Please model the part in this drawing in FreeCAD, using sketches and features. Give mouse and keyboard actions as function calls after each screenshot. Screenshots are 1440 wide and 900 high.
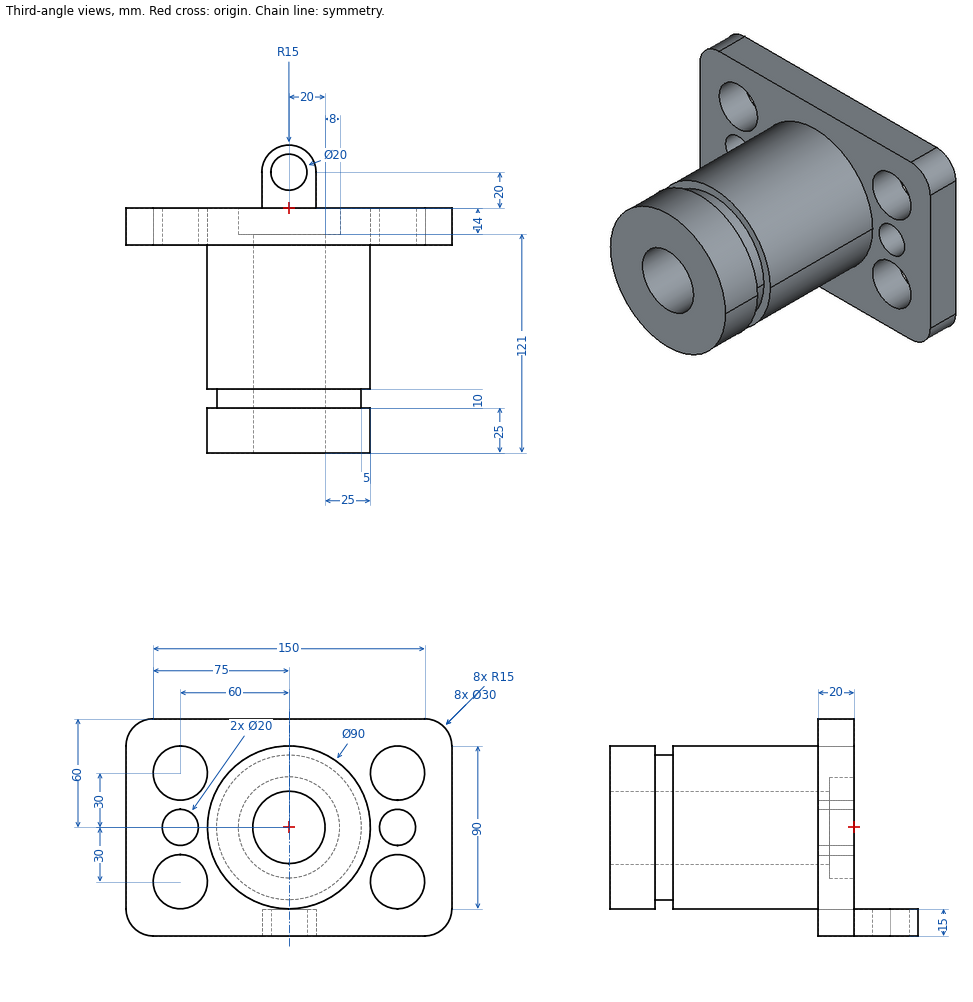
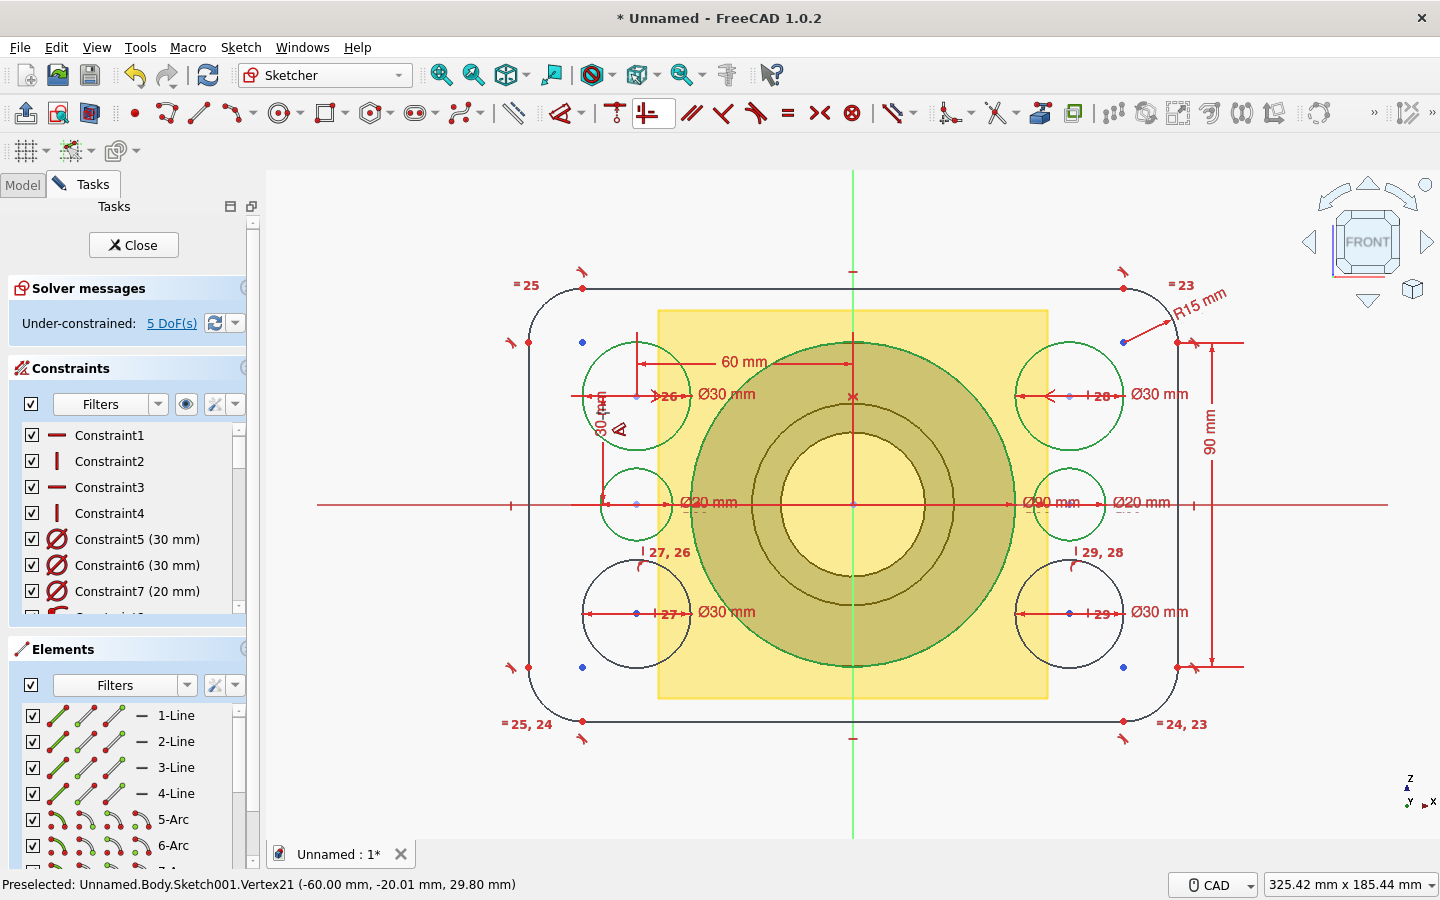
click(637, 614)
click(603, 598)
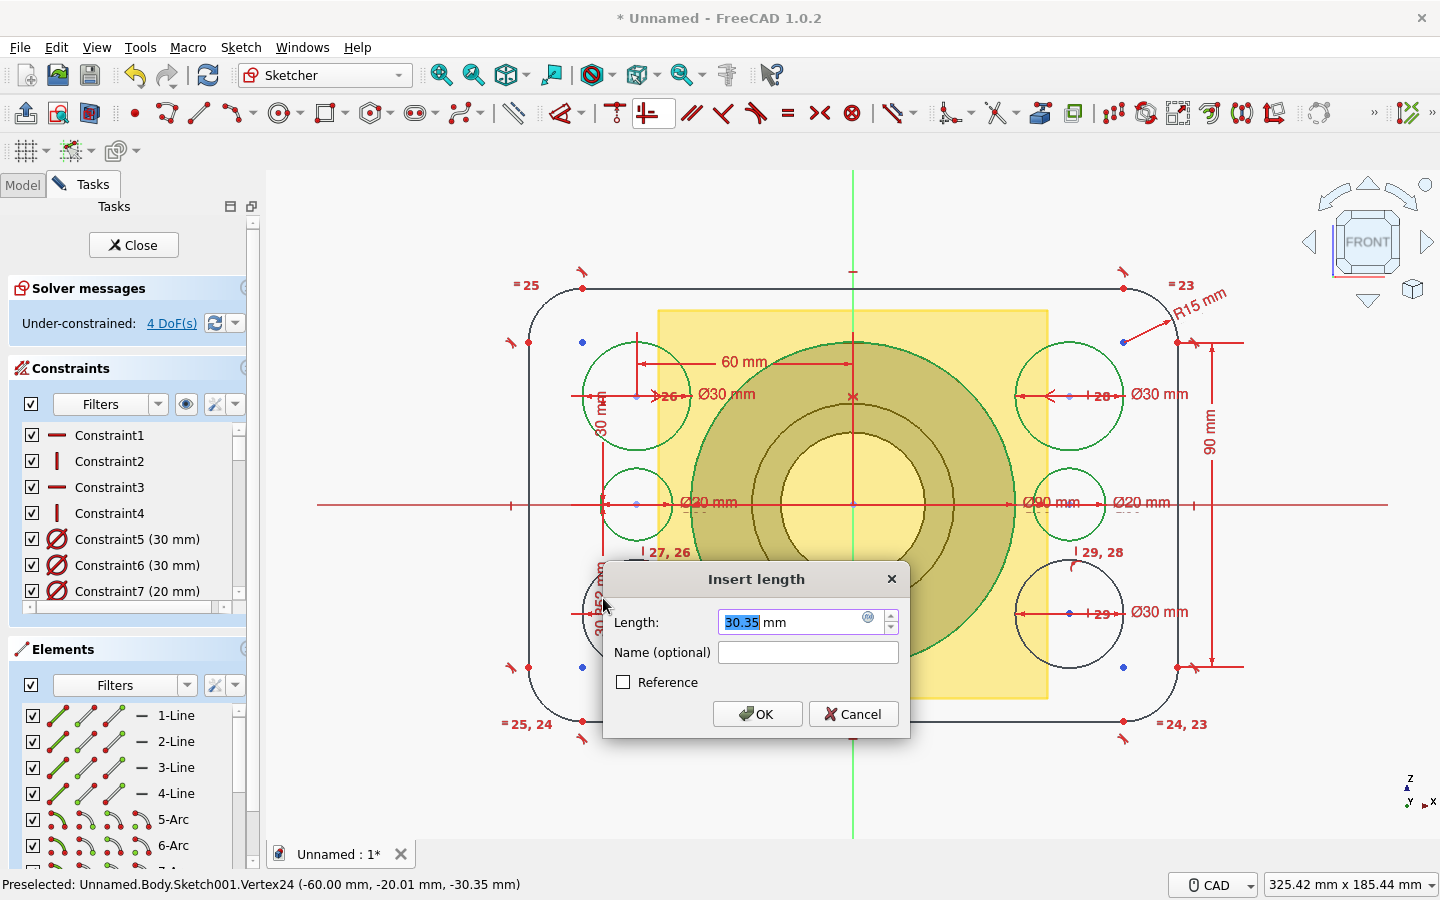
text(30)
key(Return)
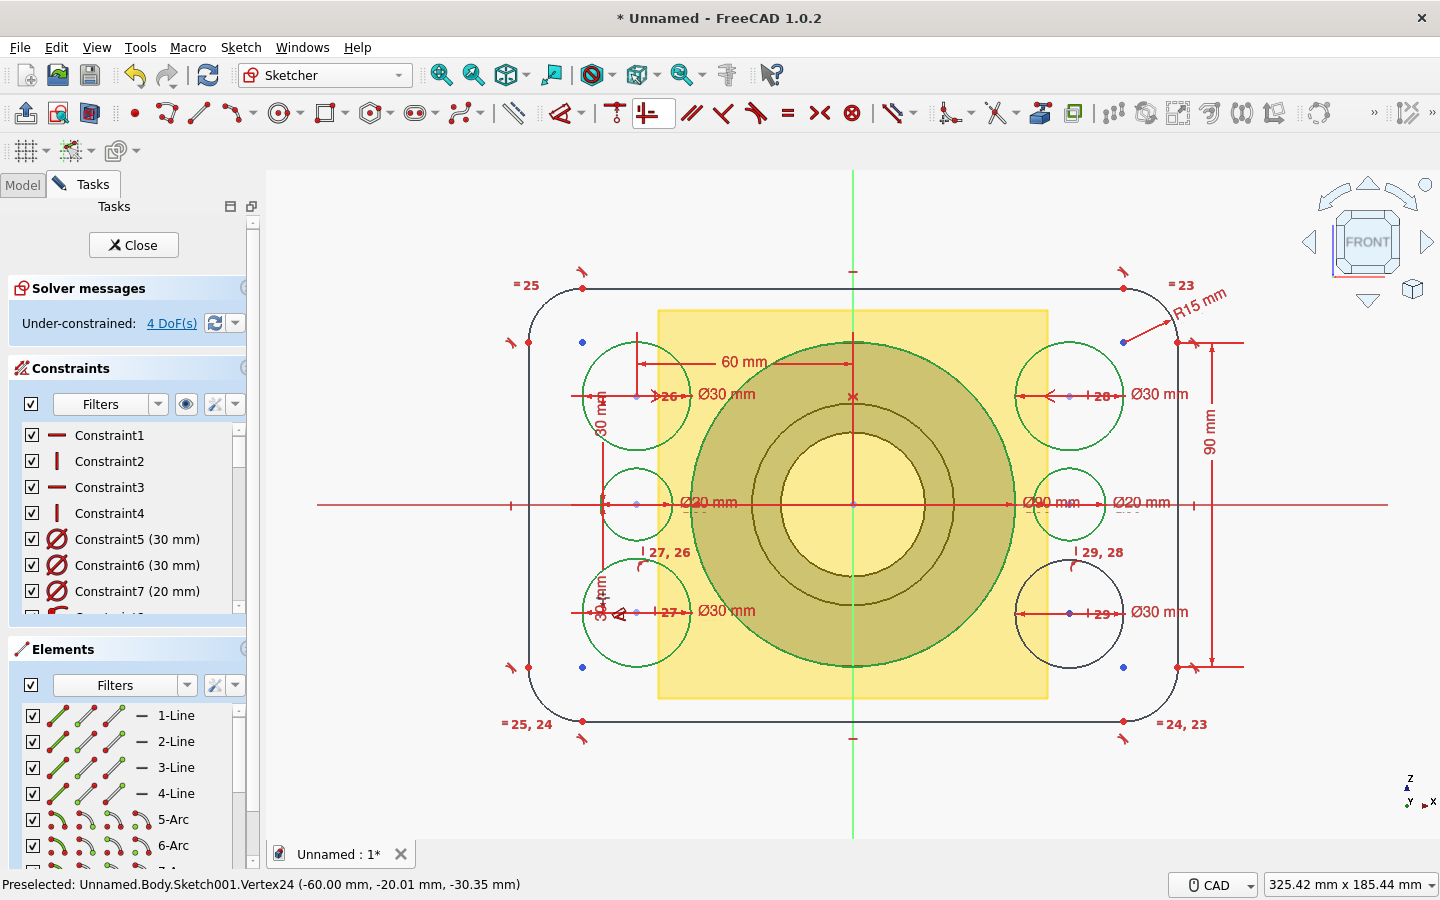
click(1069, 614)
click(1103, 598)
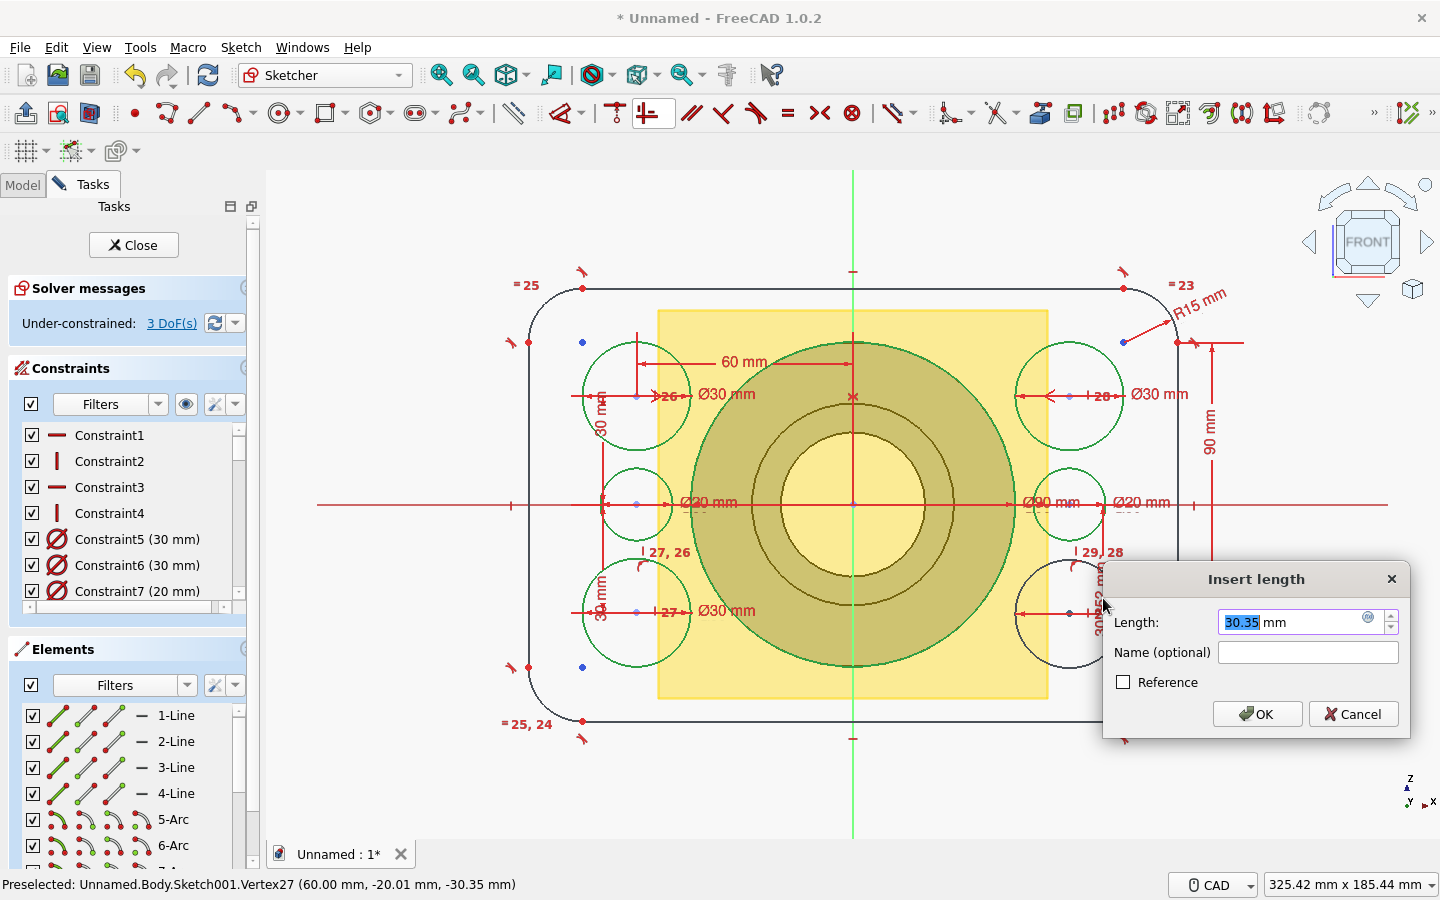
text(30)
key(Return)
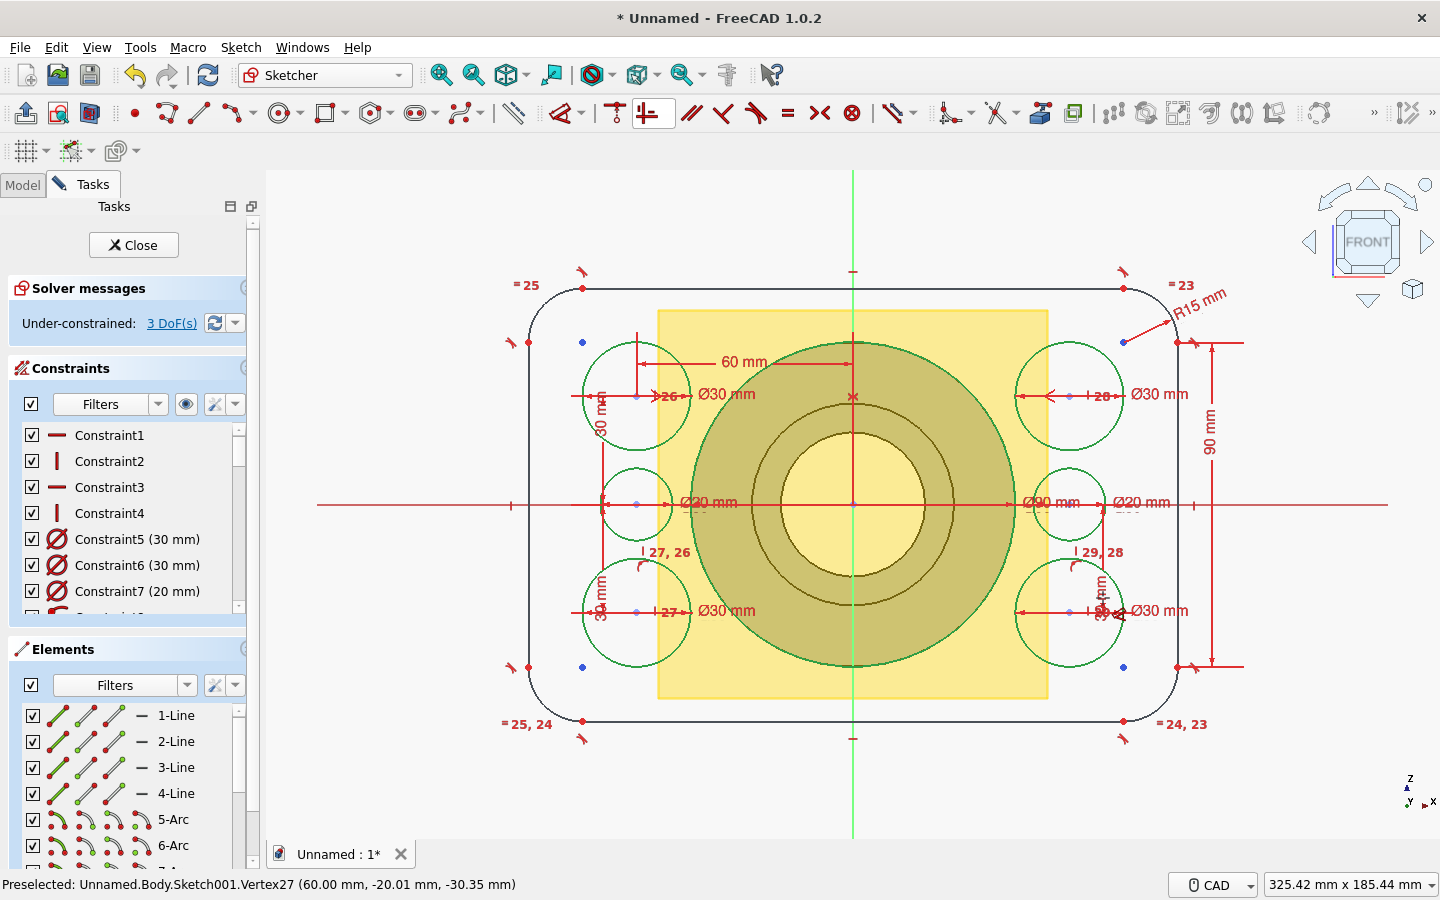
click(745, 289)
click(729, 255)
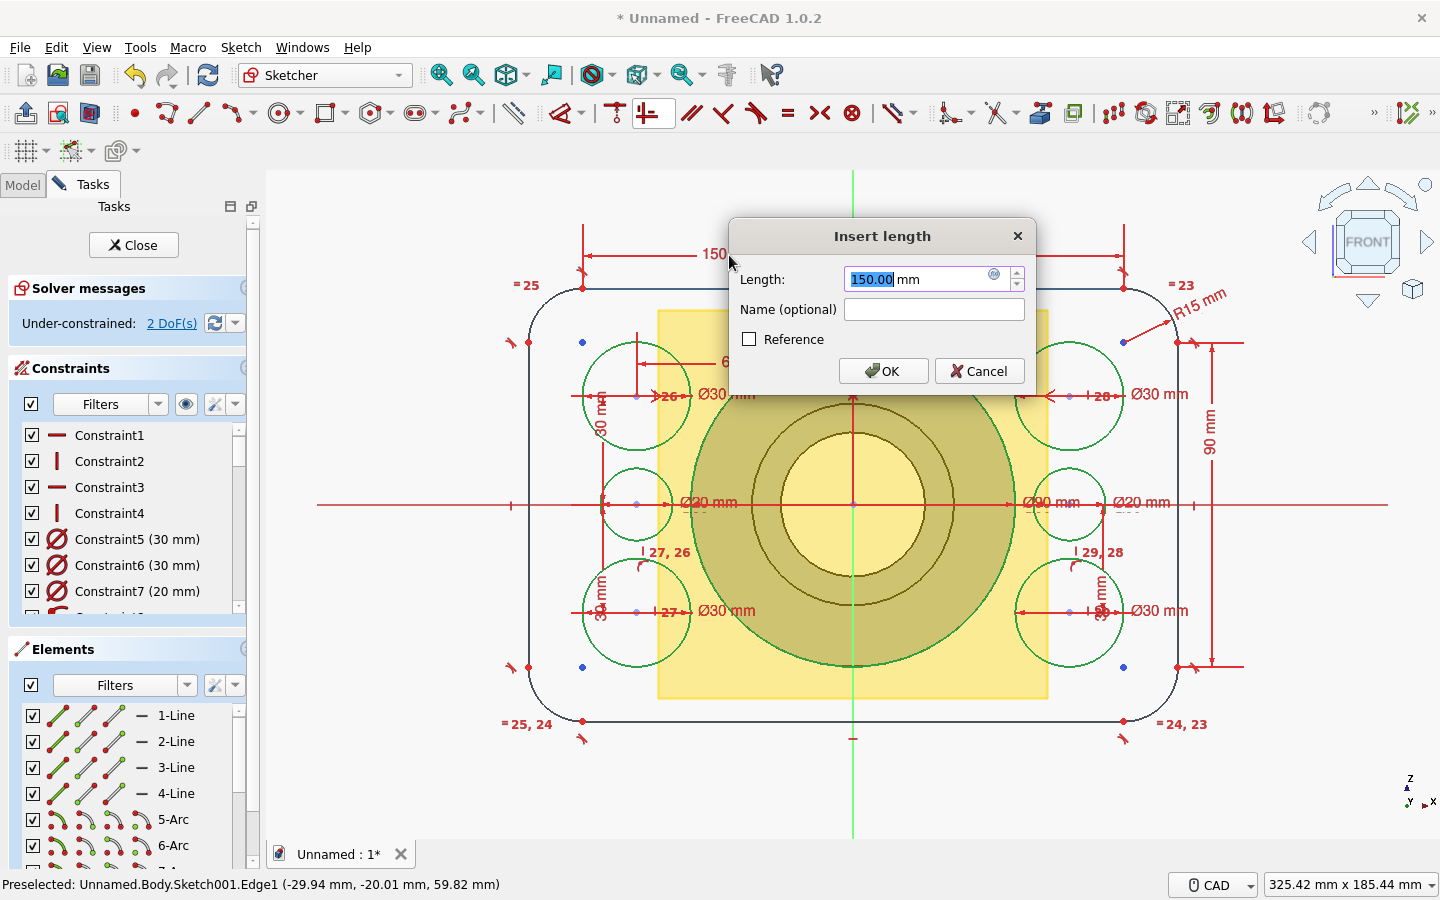
text(150)
key(Return)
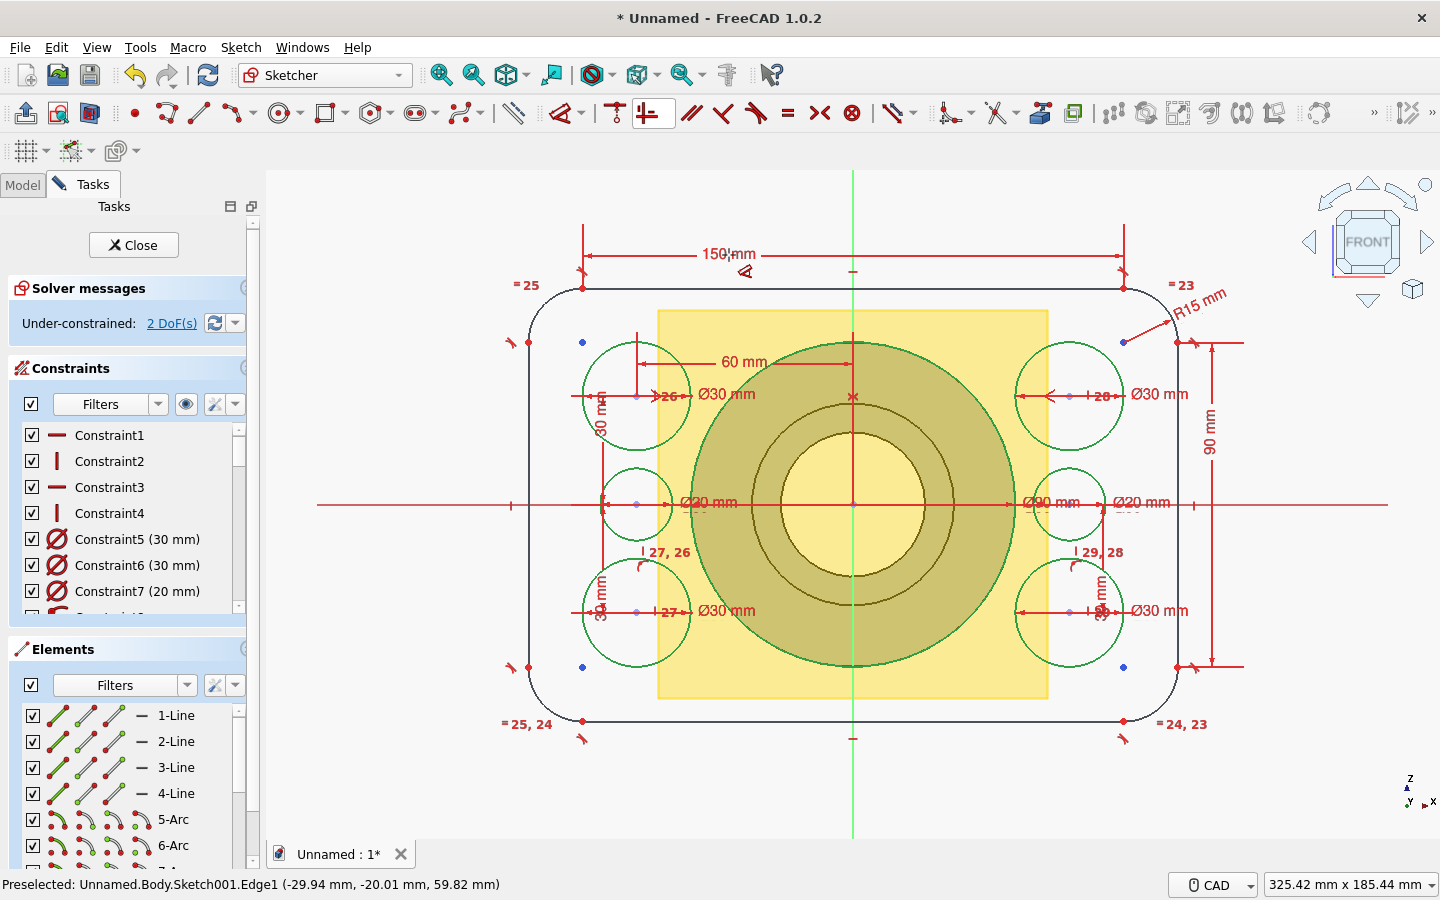
click(583, 289)
click(656, 255)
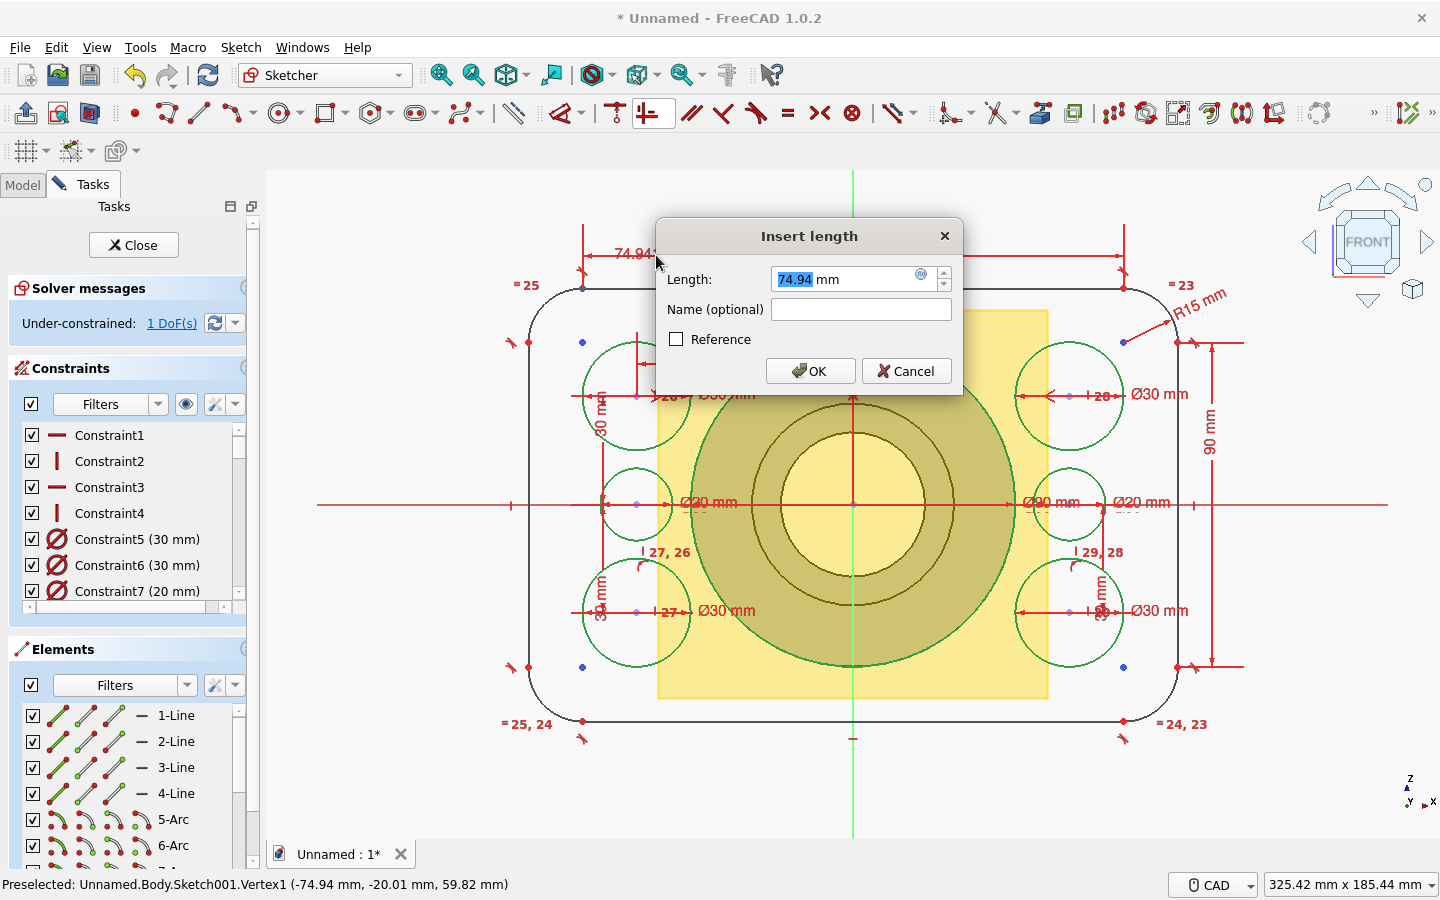
text(75)
key(Return)